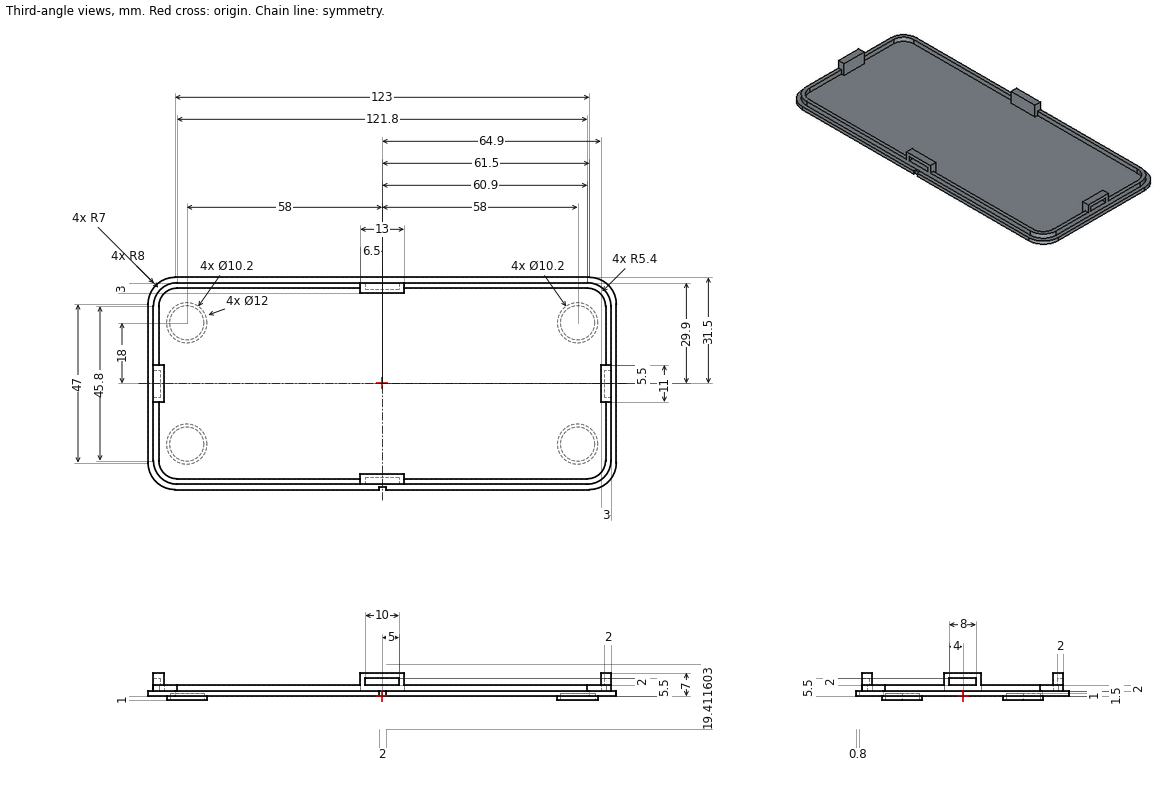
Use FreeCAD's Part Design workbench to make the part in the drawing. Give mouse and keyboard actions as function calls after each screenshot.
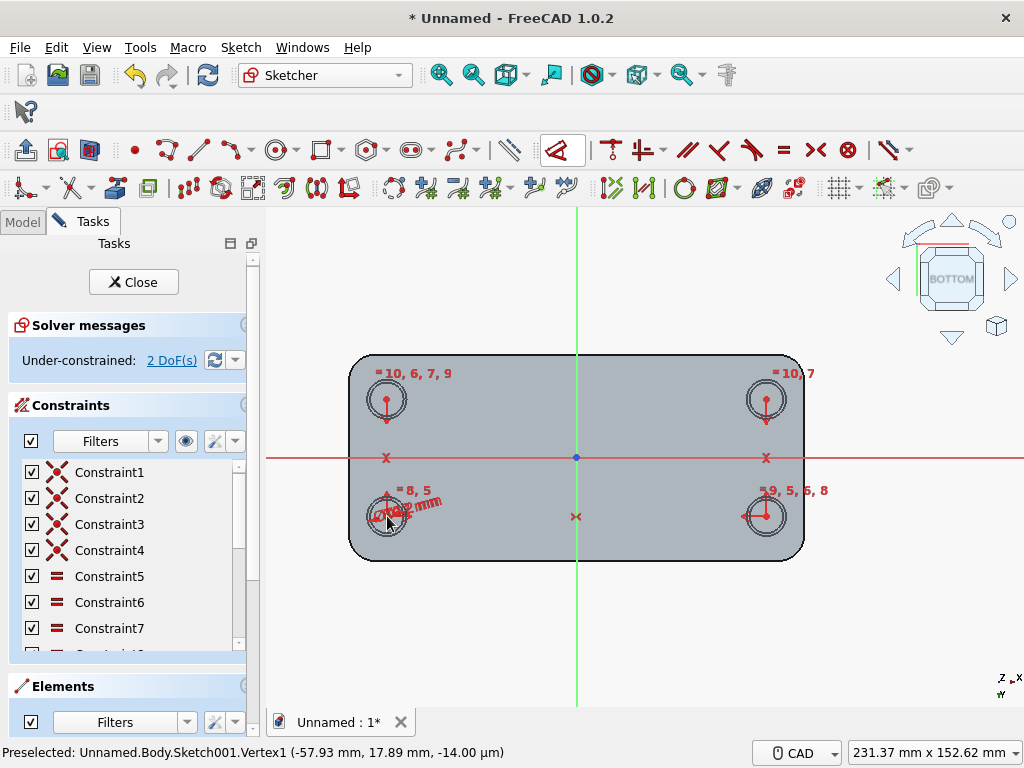
key(l)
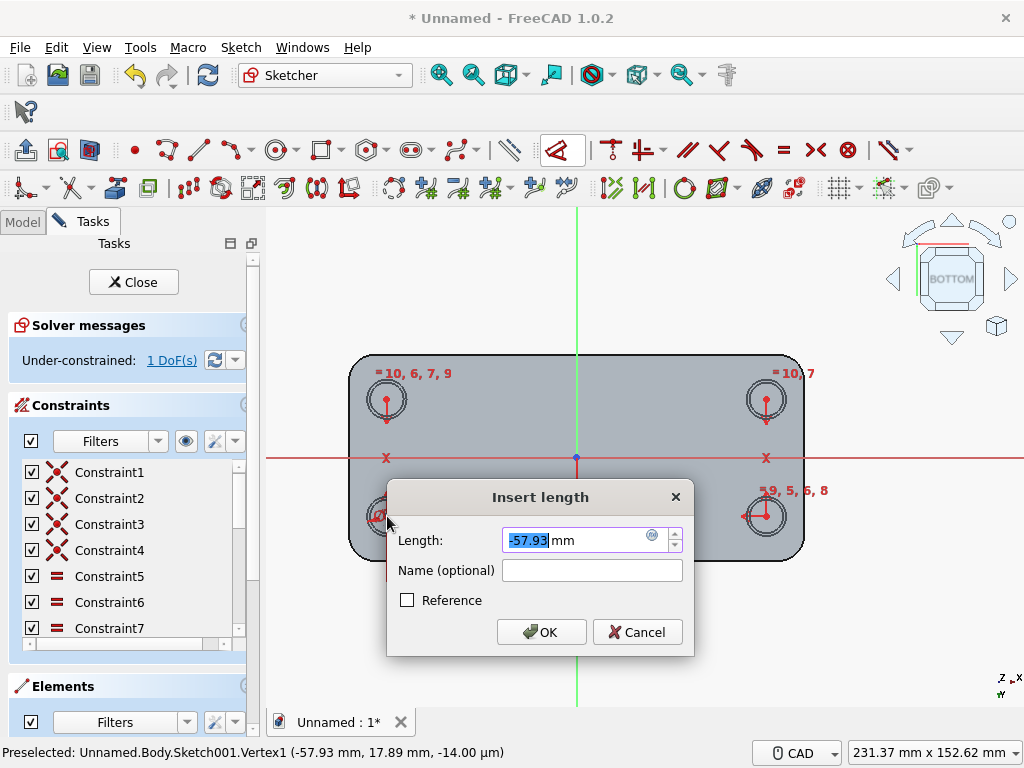
text(-58)
key(Return)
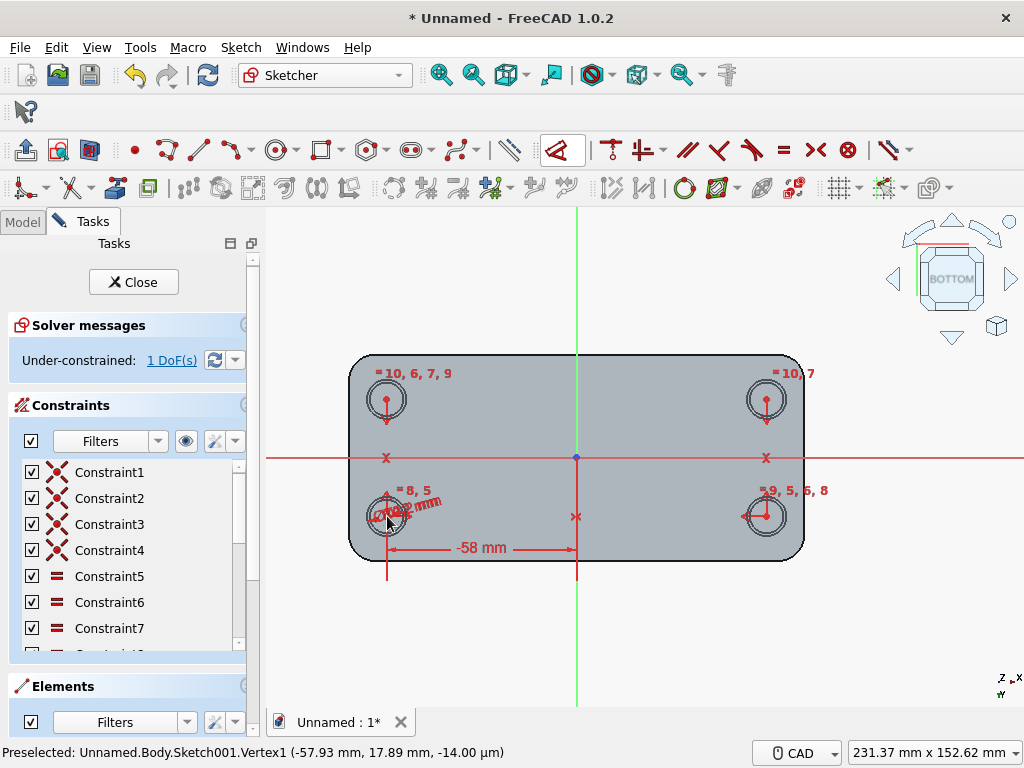
click(387, 516)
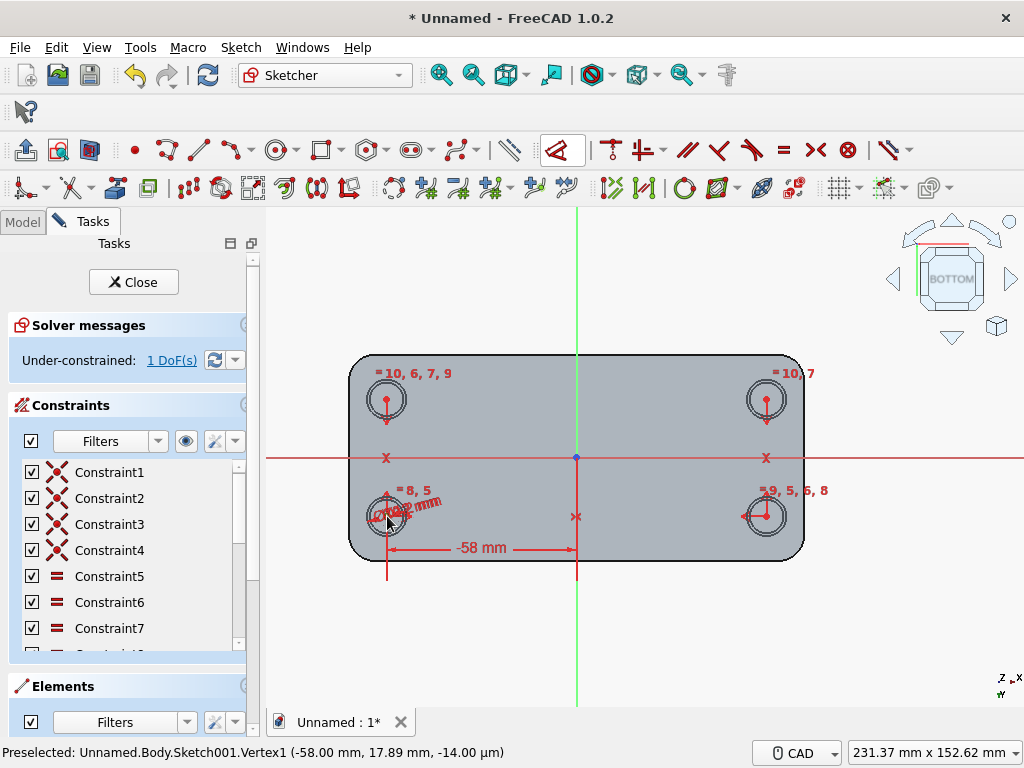
key(i)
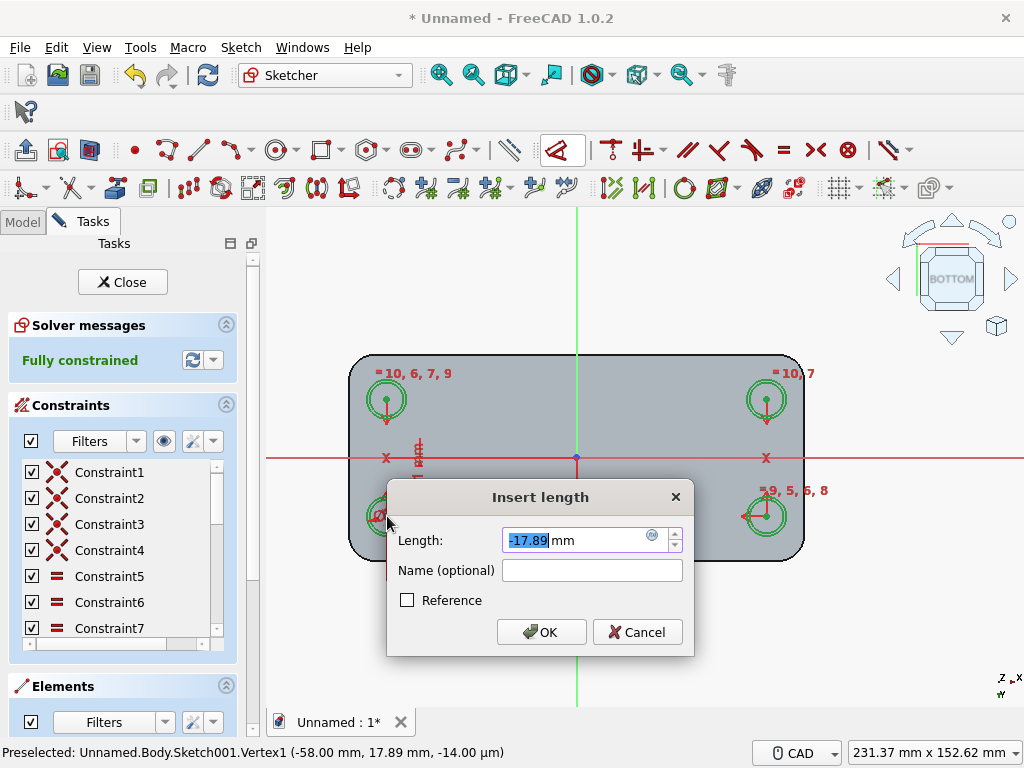
text(-18)
key(Return)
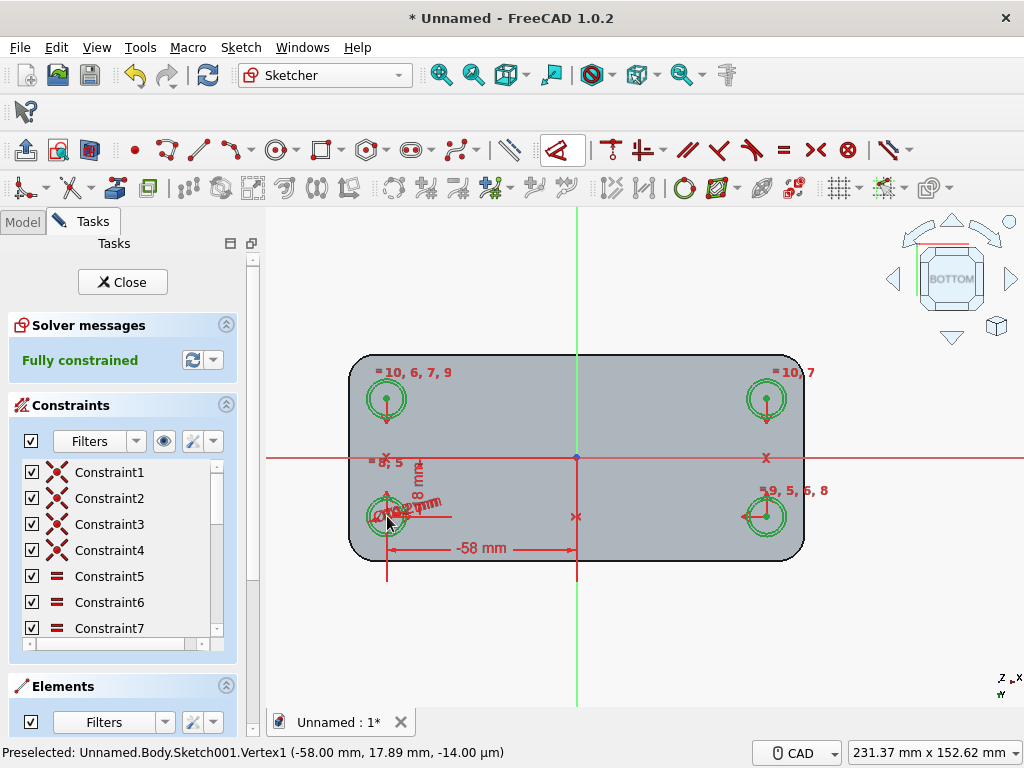
click(123, 282)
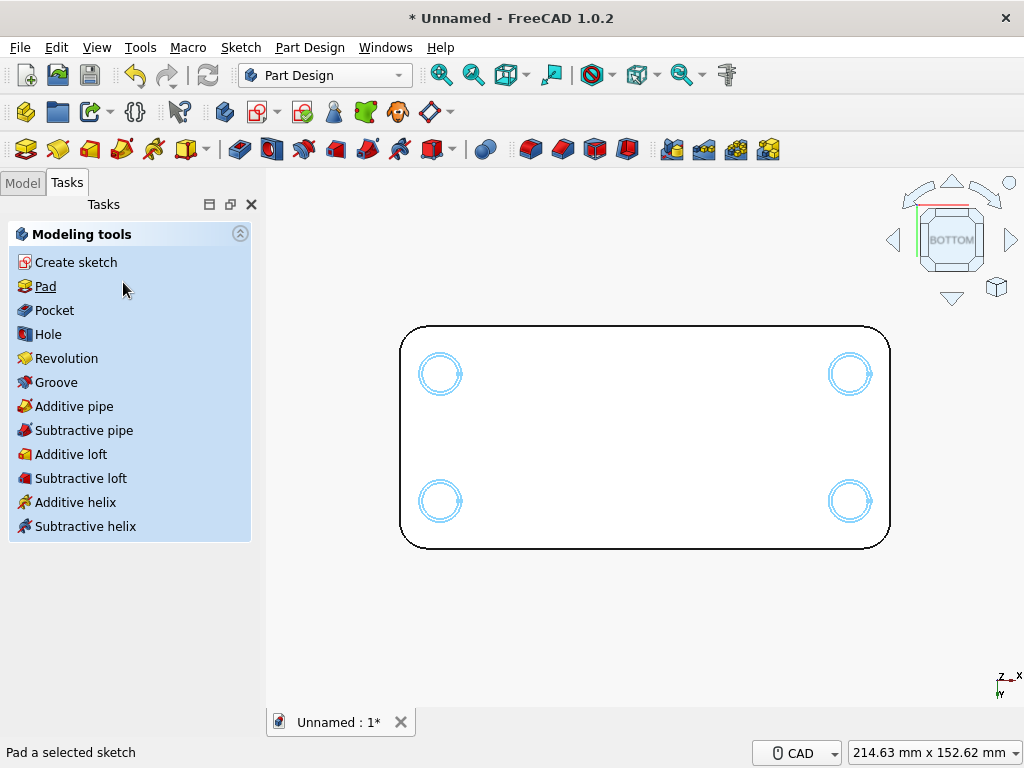
click(26, 150)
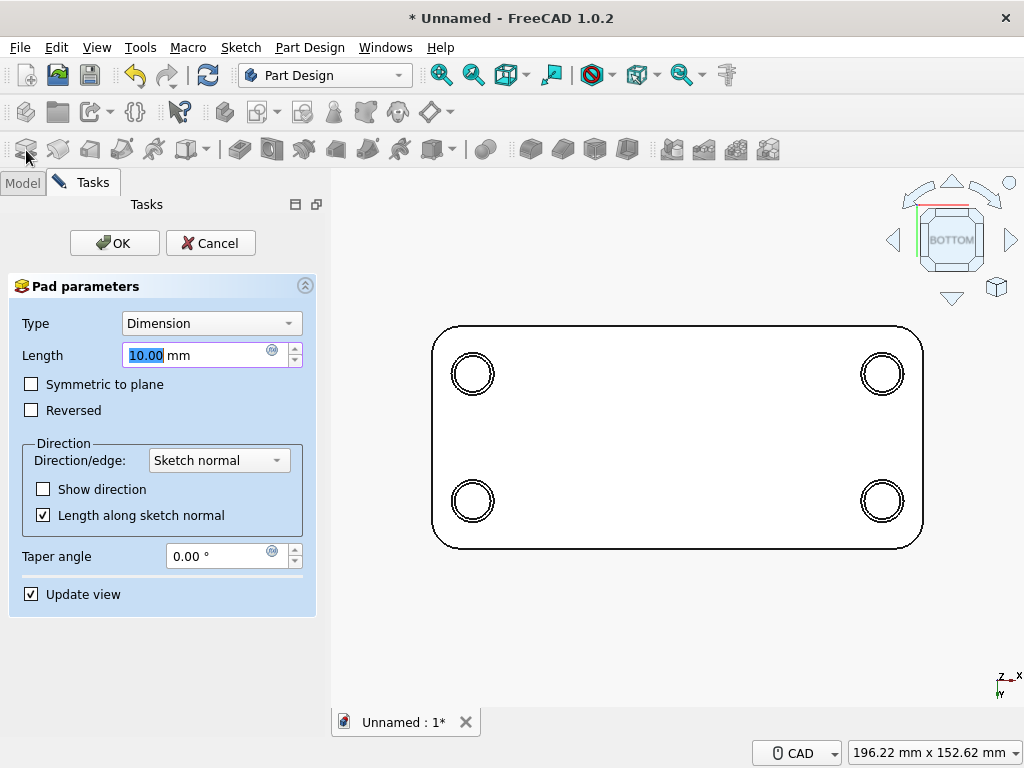
text(1)
key(Tab)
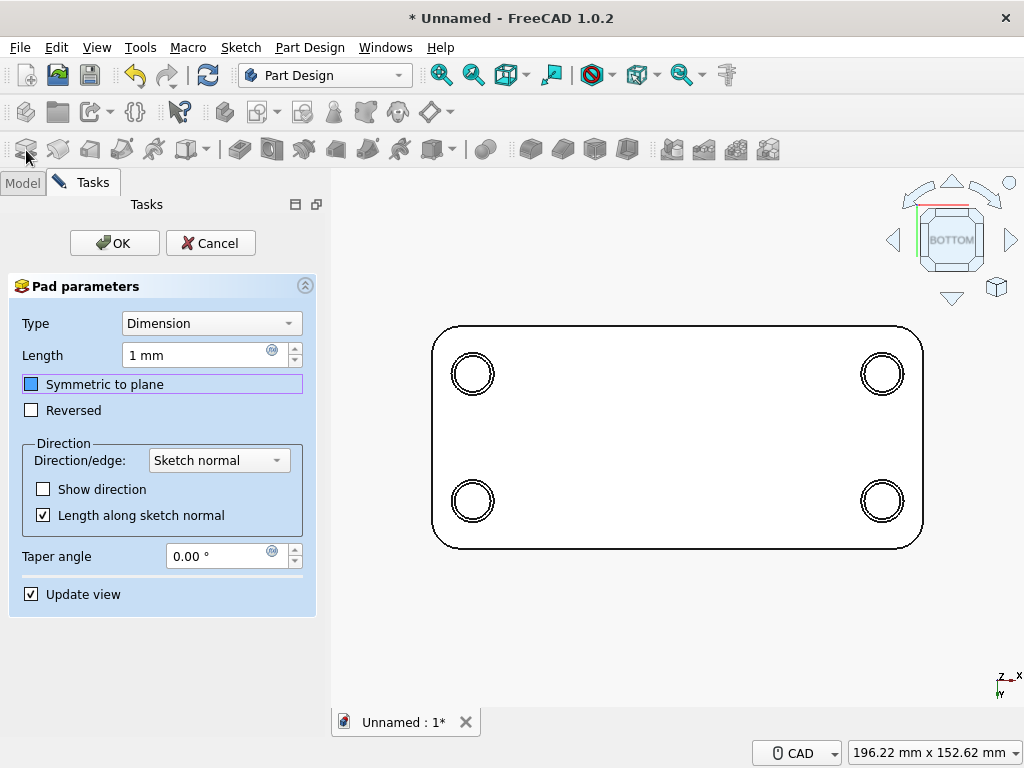
click(115, 243)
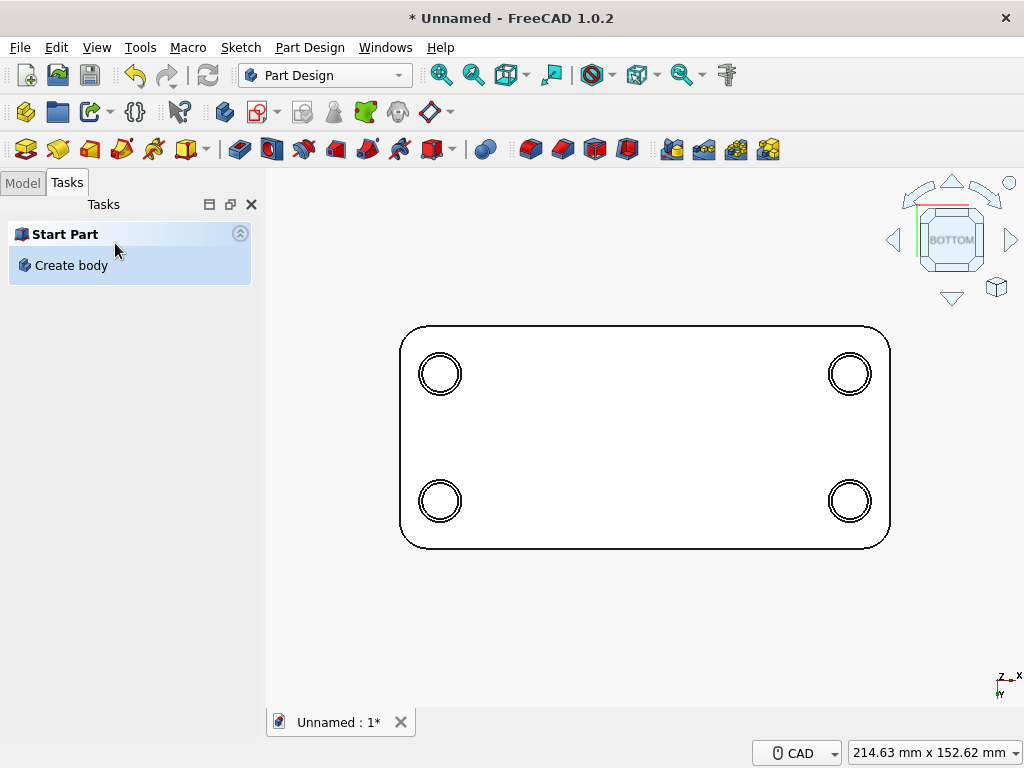
key(0)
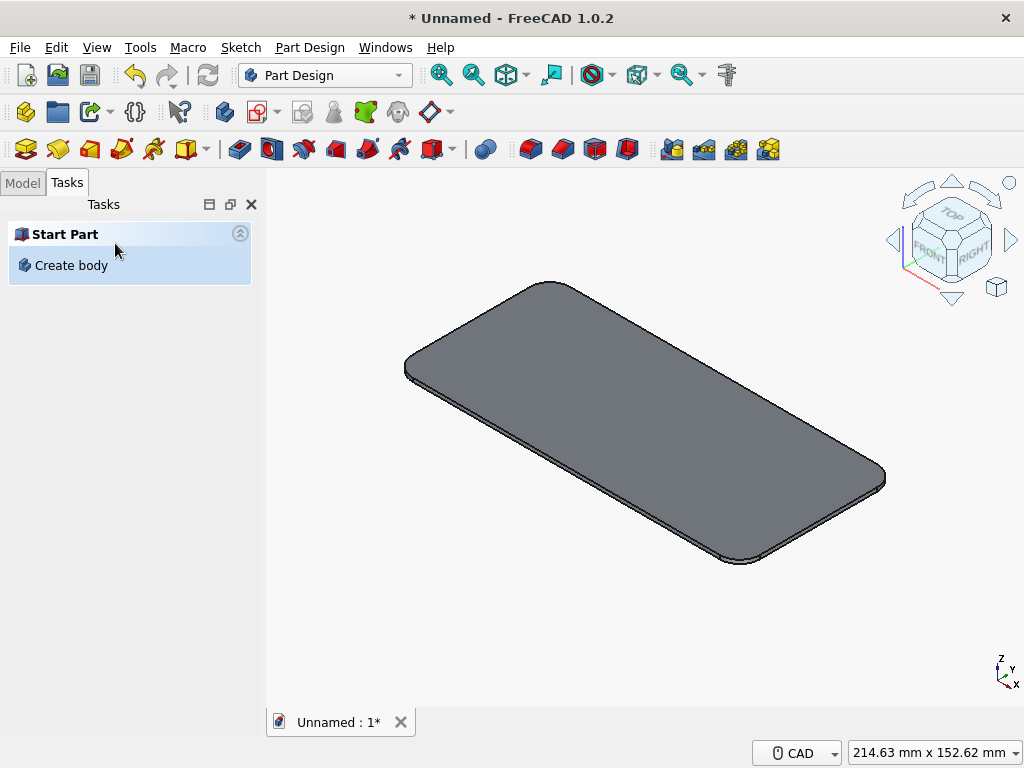
click(695, 449)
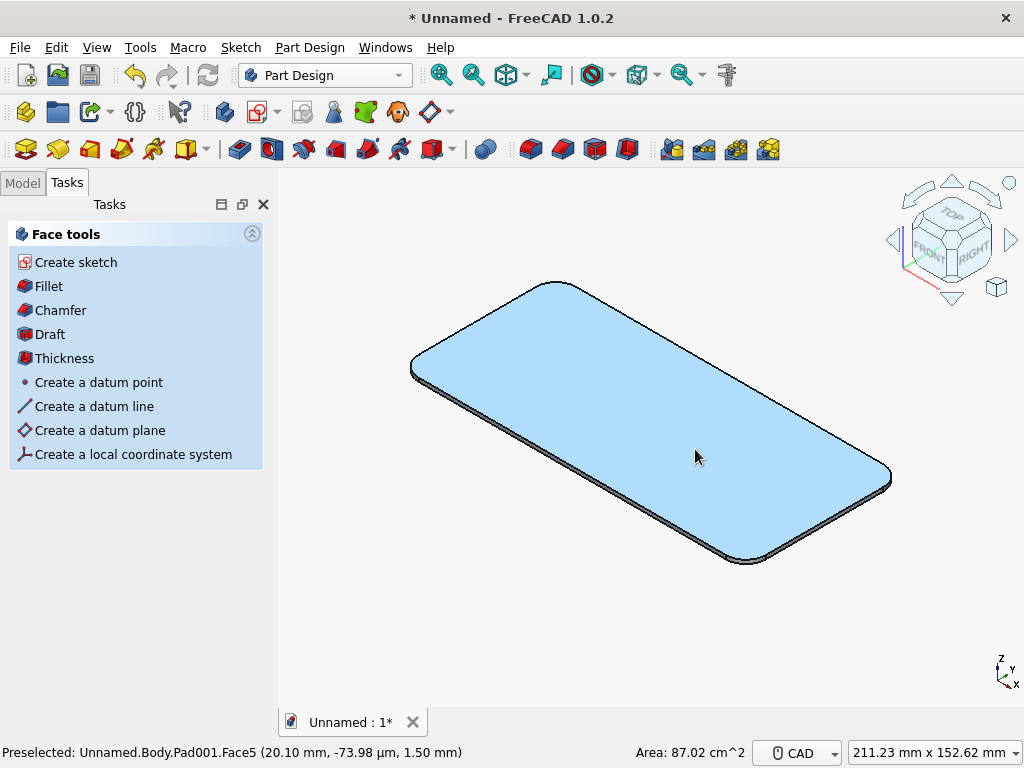
click(258, 112)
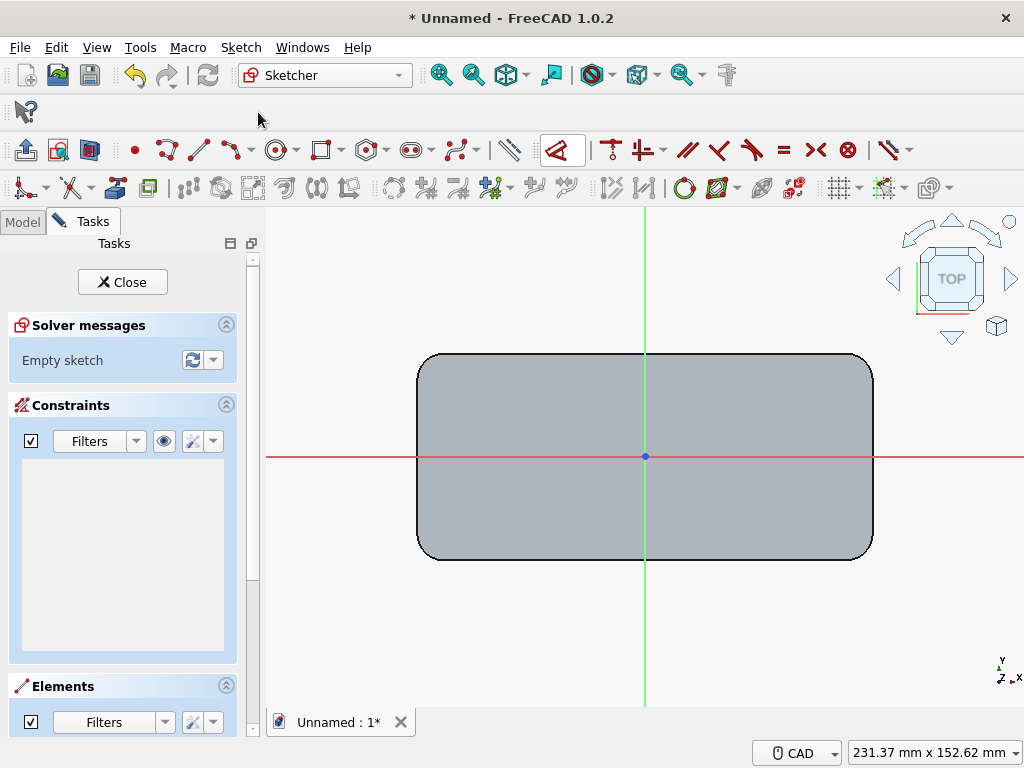
scroll(294, 457, down, 1)